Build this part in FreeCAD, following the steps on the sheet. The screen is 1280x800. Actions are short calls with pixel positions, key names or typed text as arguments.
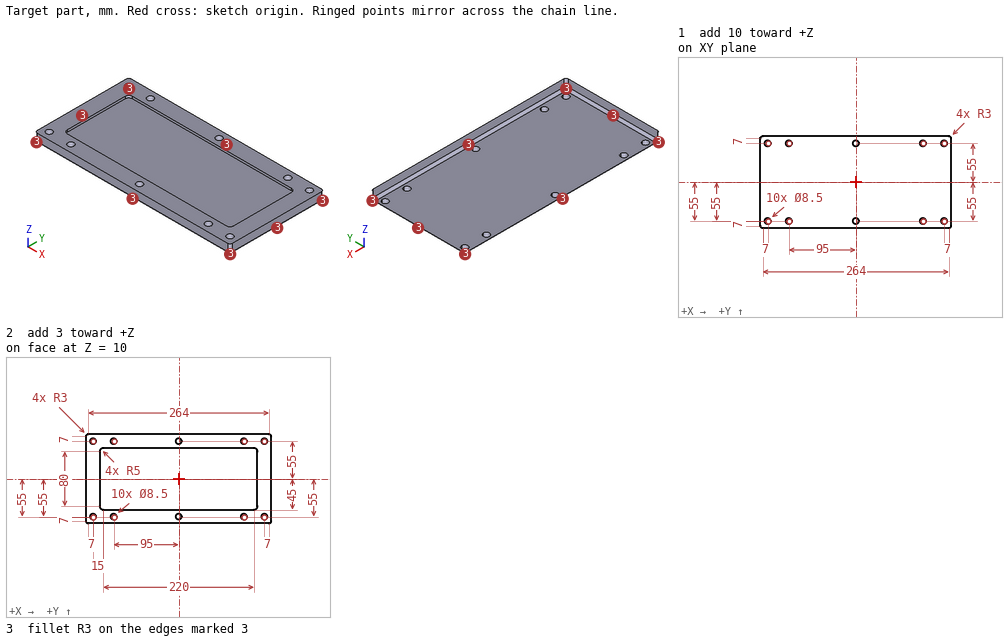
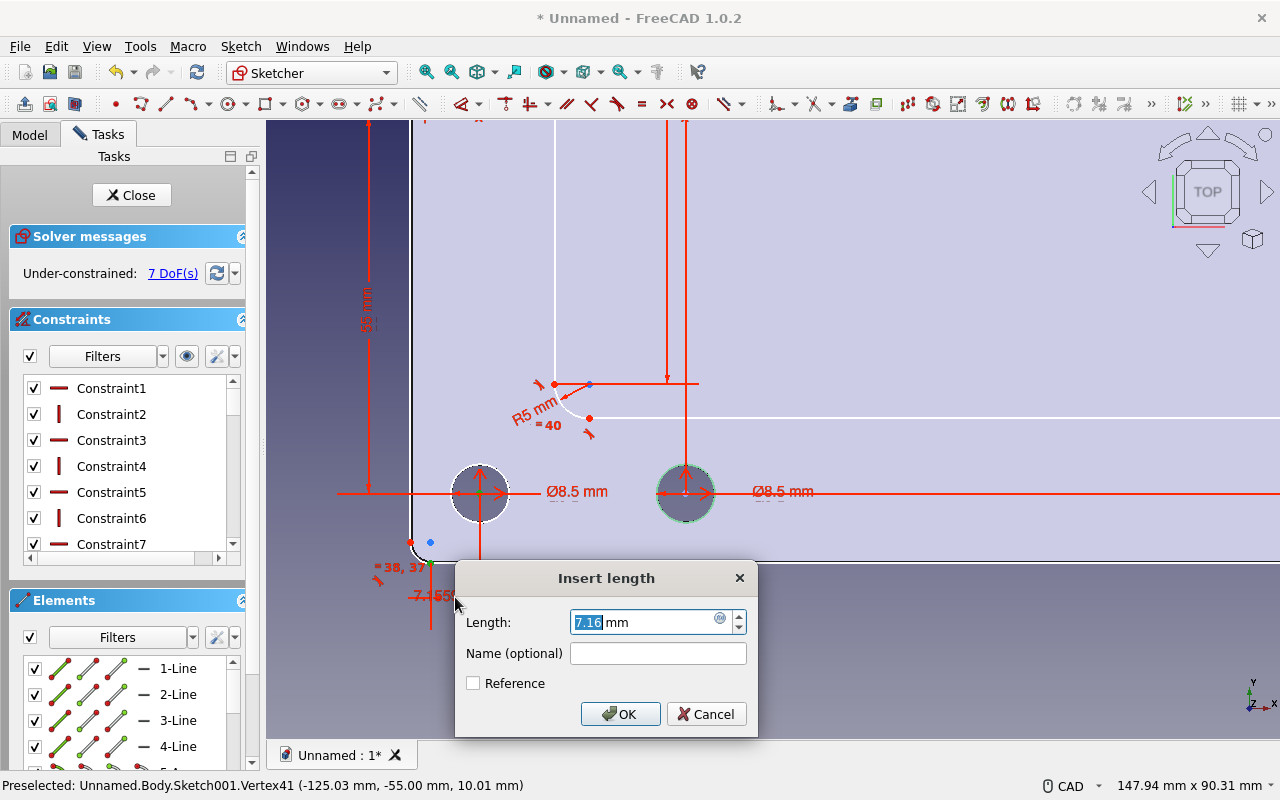
text(7)
key(Return)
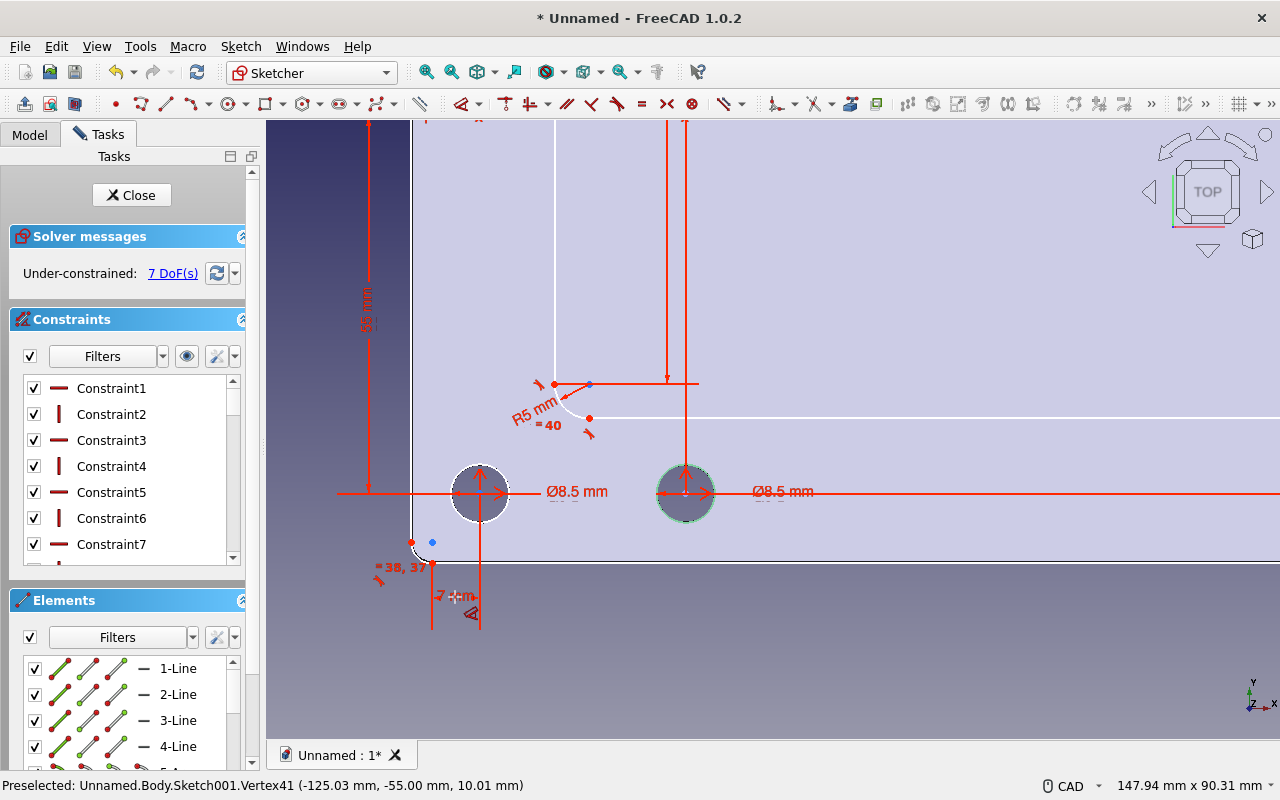
click(411, 543)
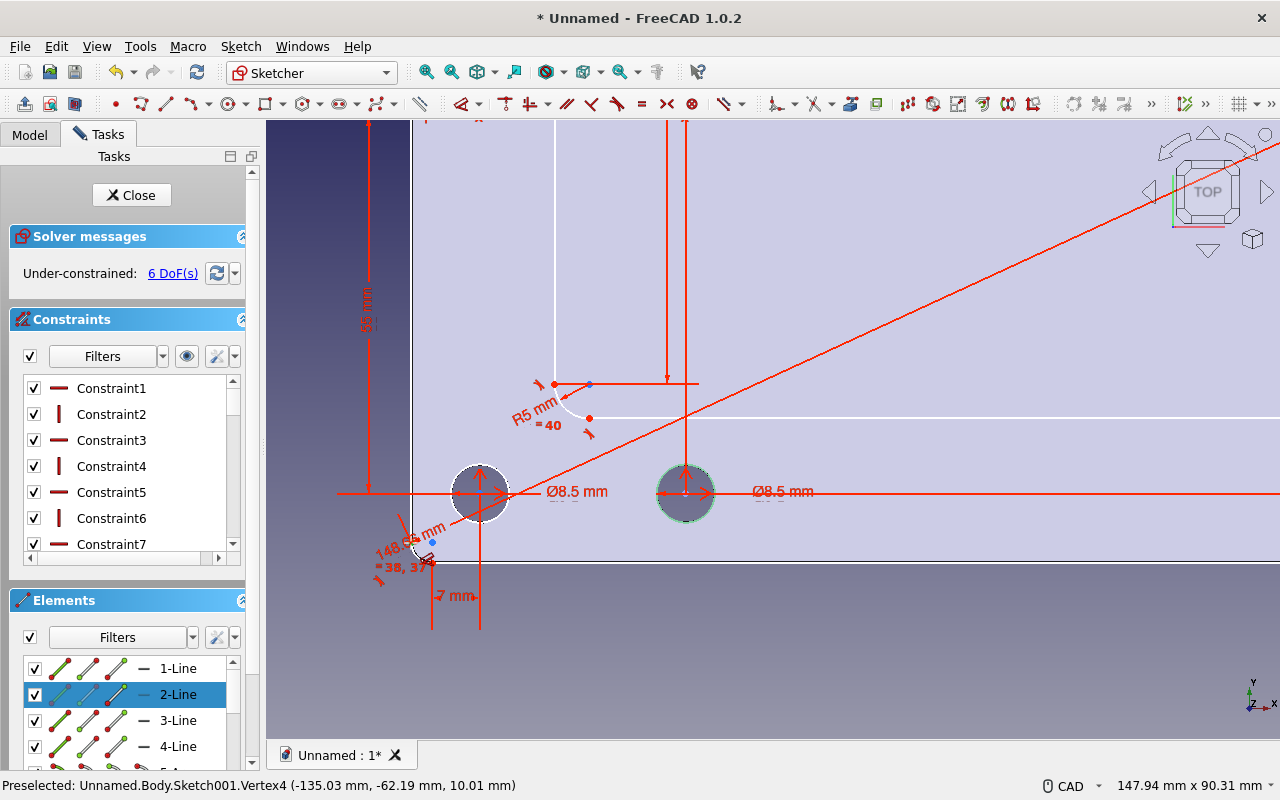
click(480, 494)
click(377, 518)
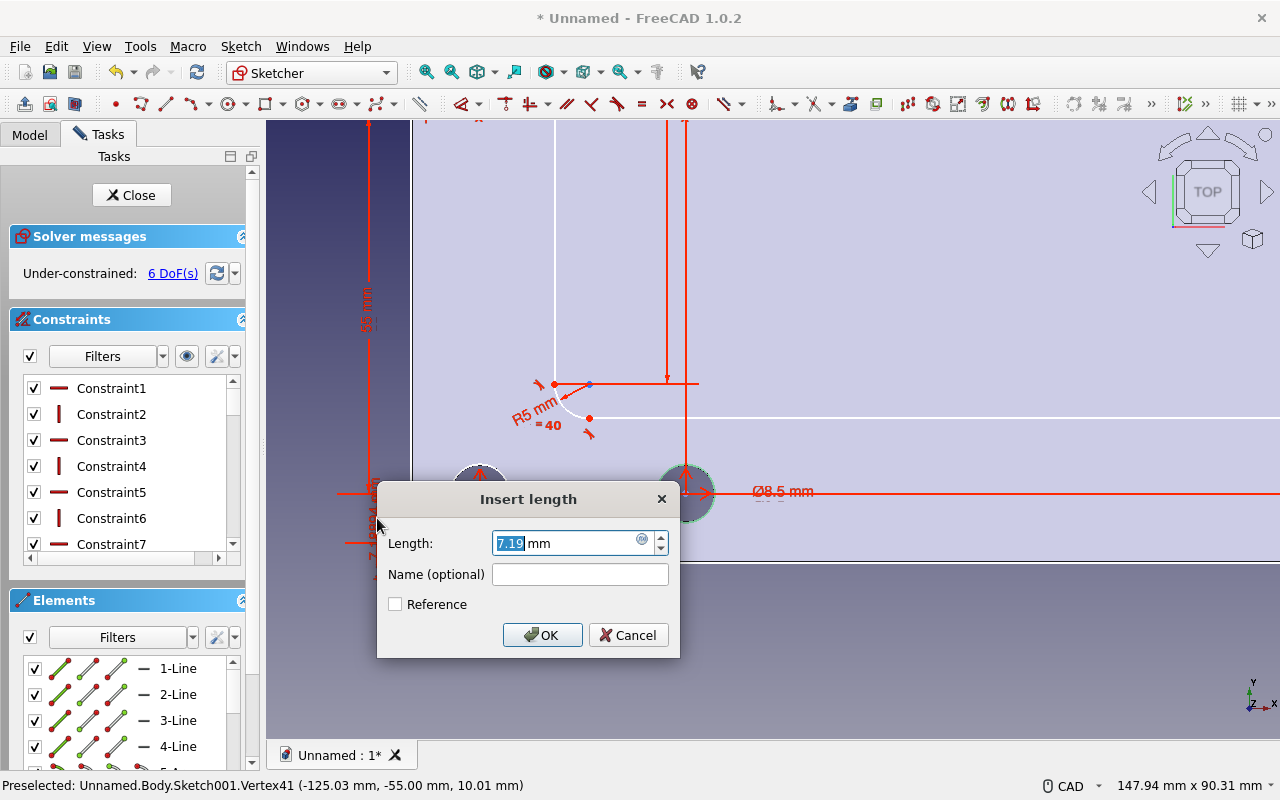
text(7)
key(Return)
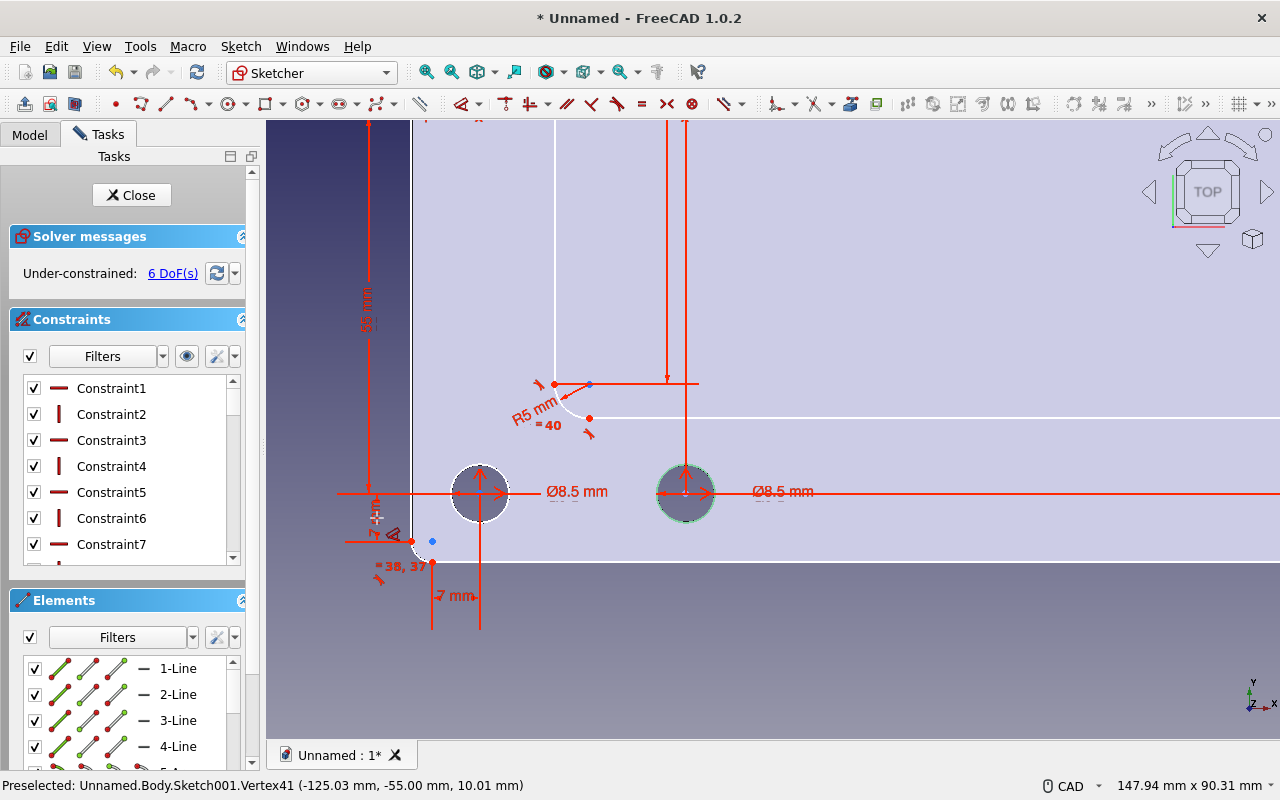
scroll(432, 564, down, 6)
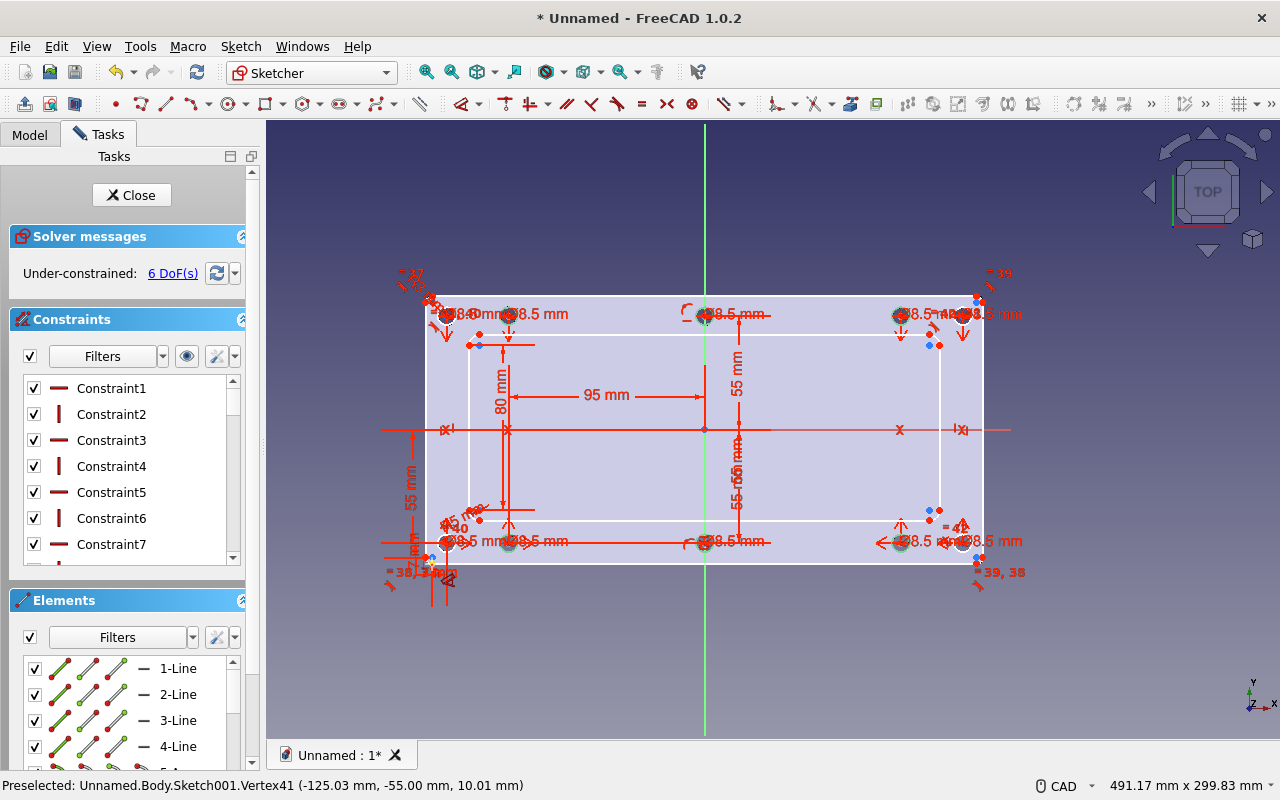
scroll(977, 564, up, 6)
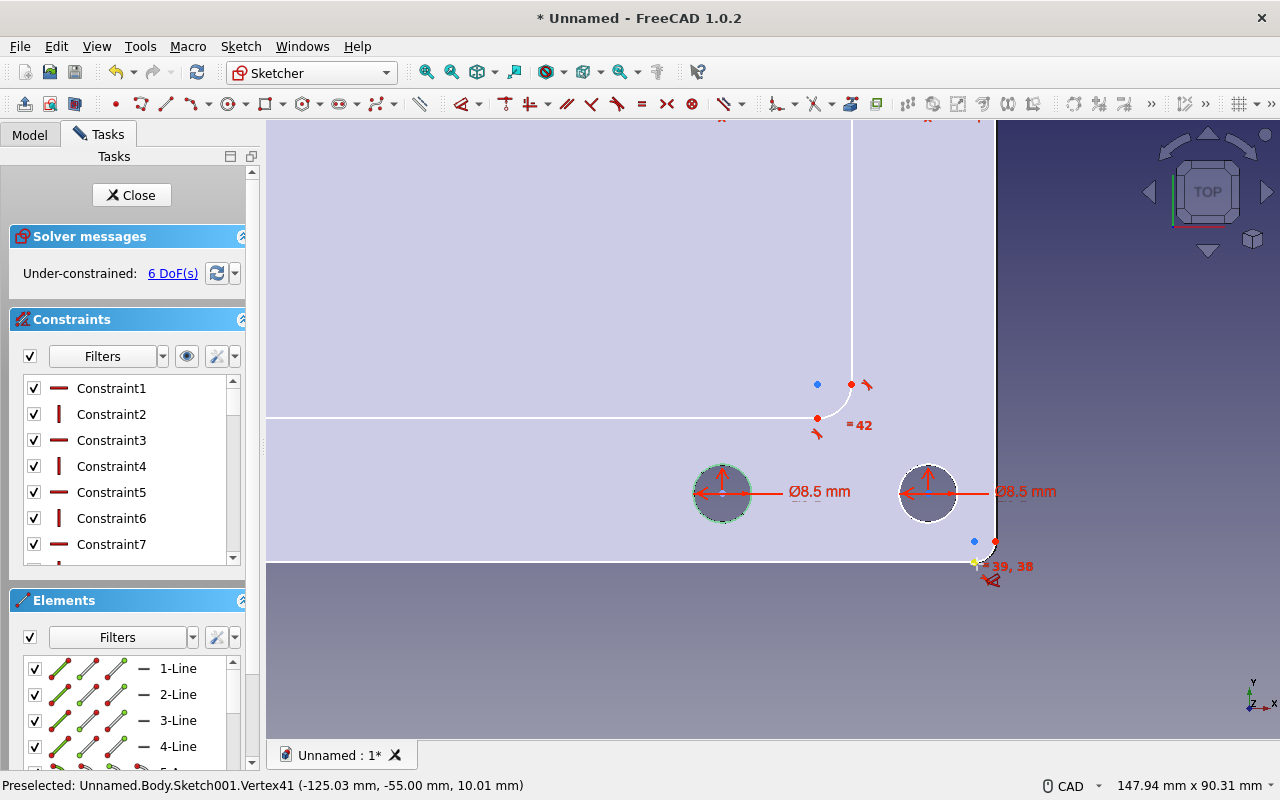
click(975, 562)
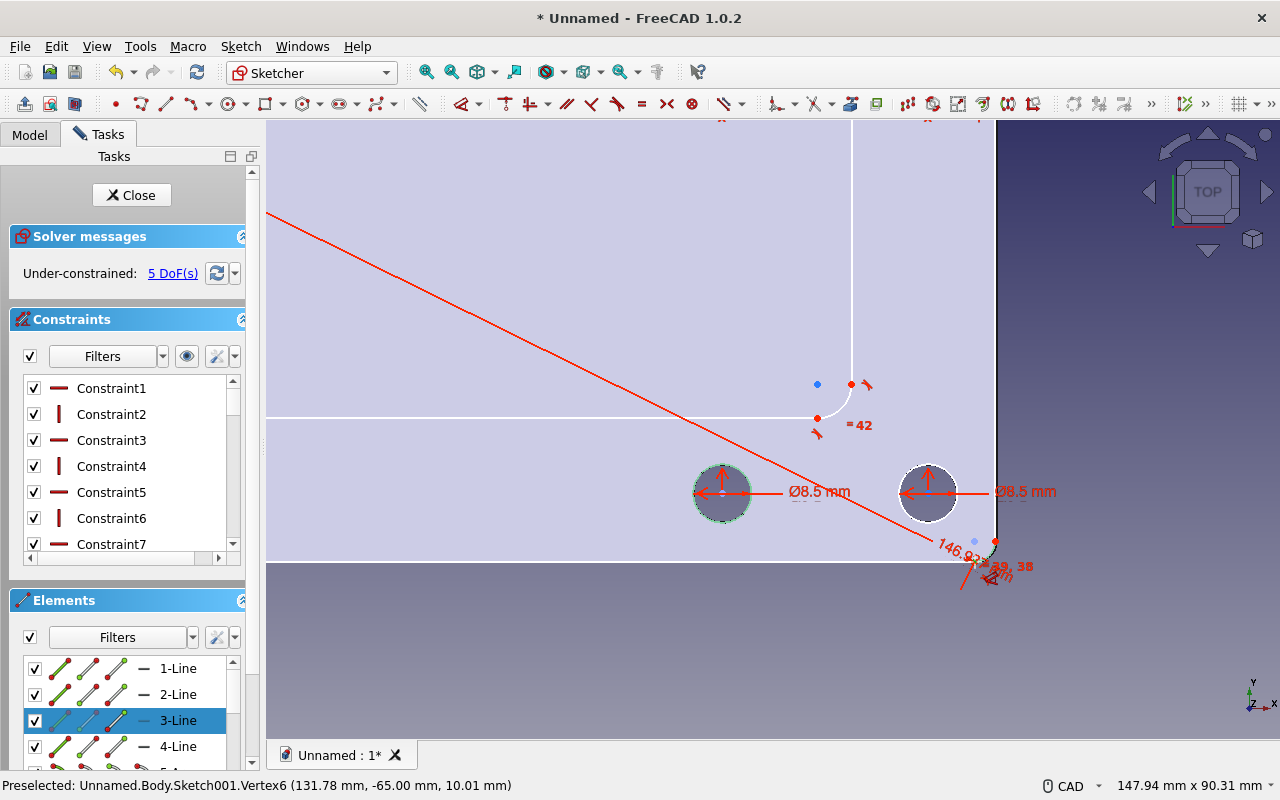
click(928, 494)
click(951, 596)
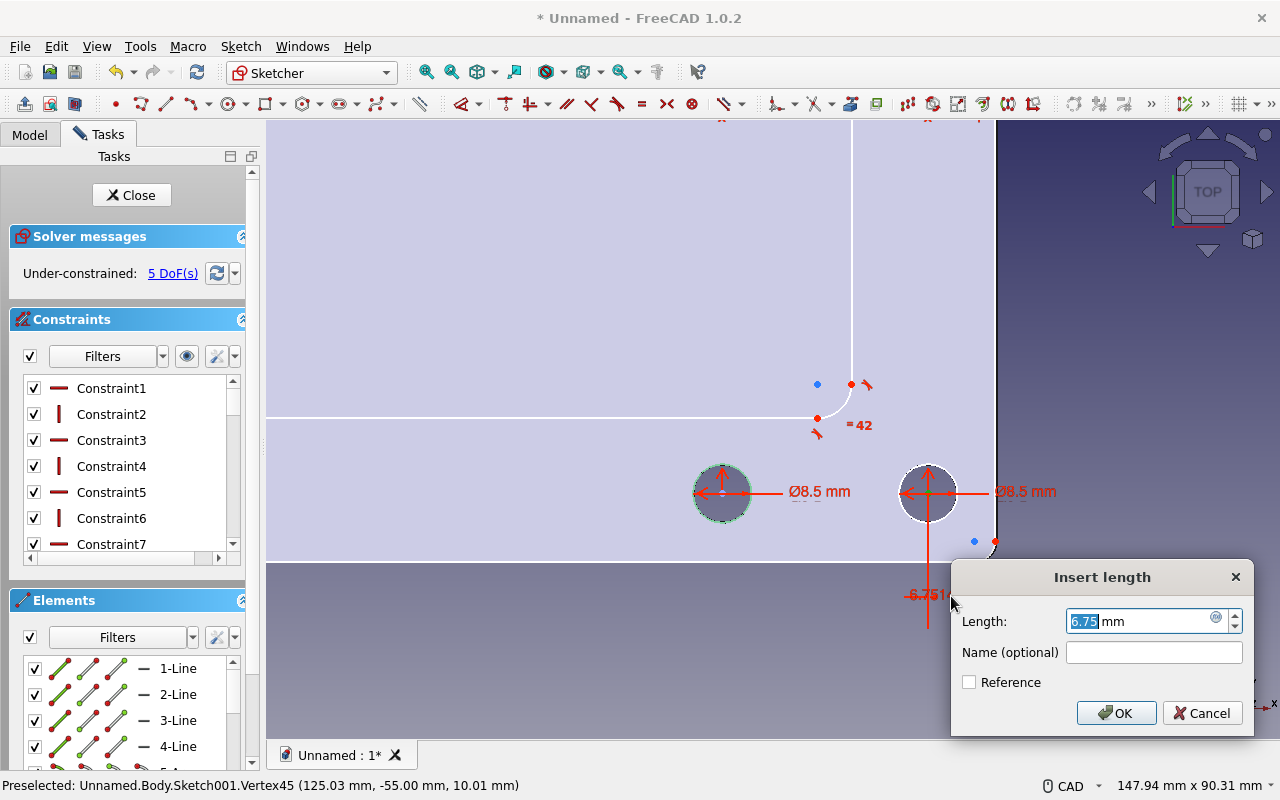
text(7)
key(Return)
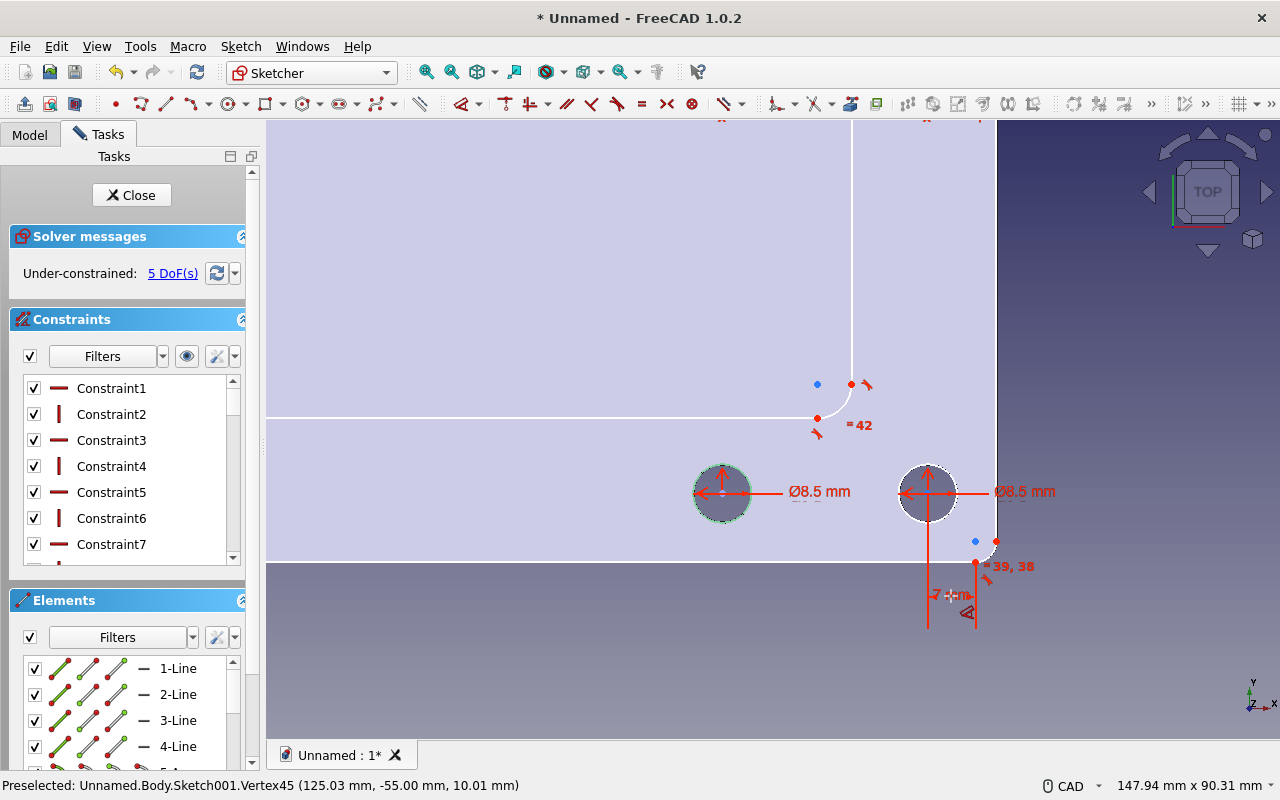
scroll(977, 564, down, 6)